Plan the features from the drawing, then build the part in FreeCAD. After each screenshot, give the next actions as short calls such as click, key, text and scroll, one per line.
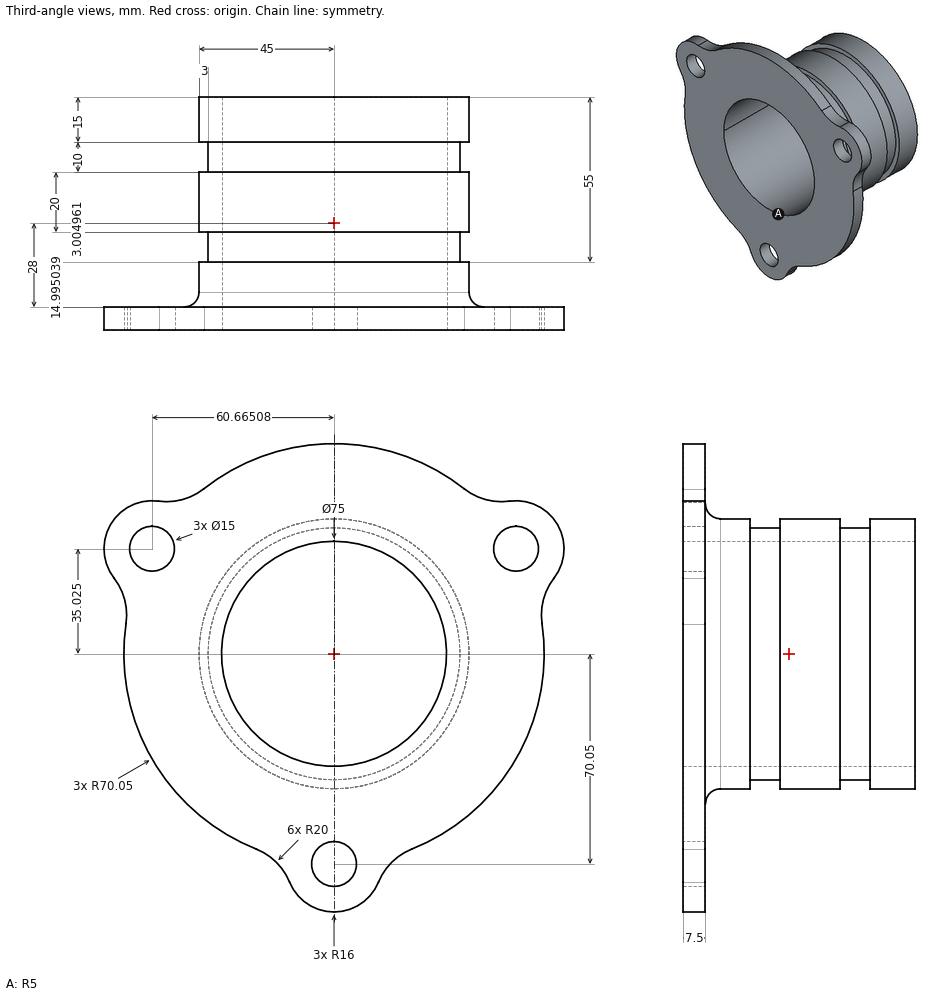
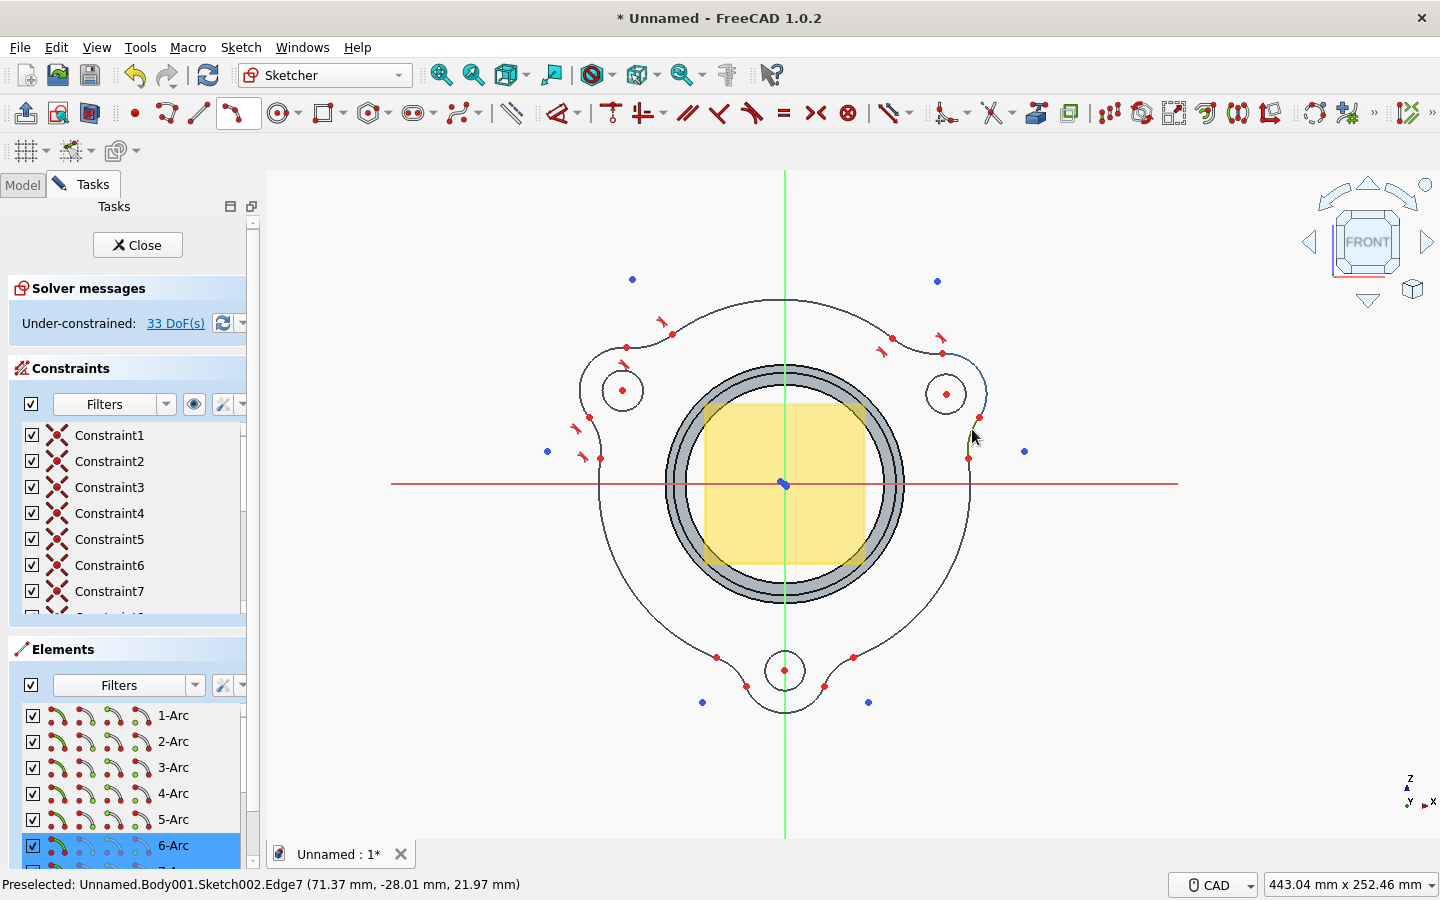
key(t)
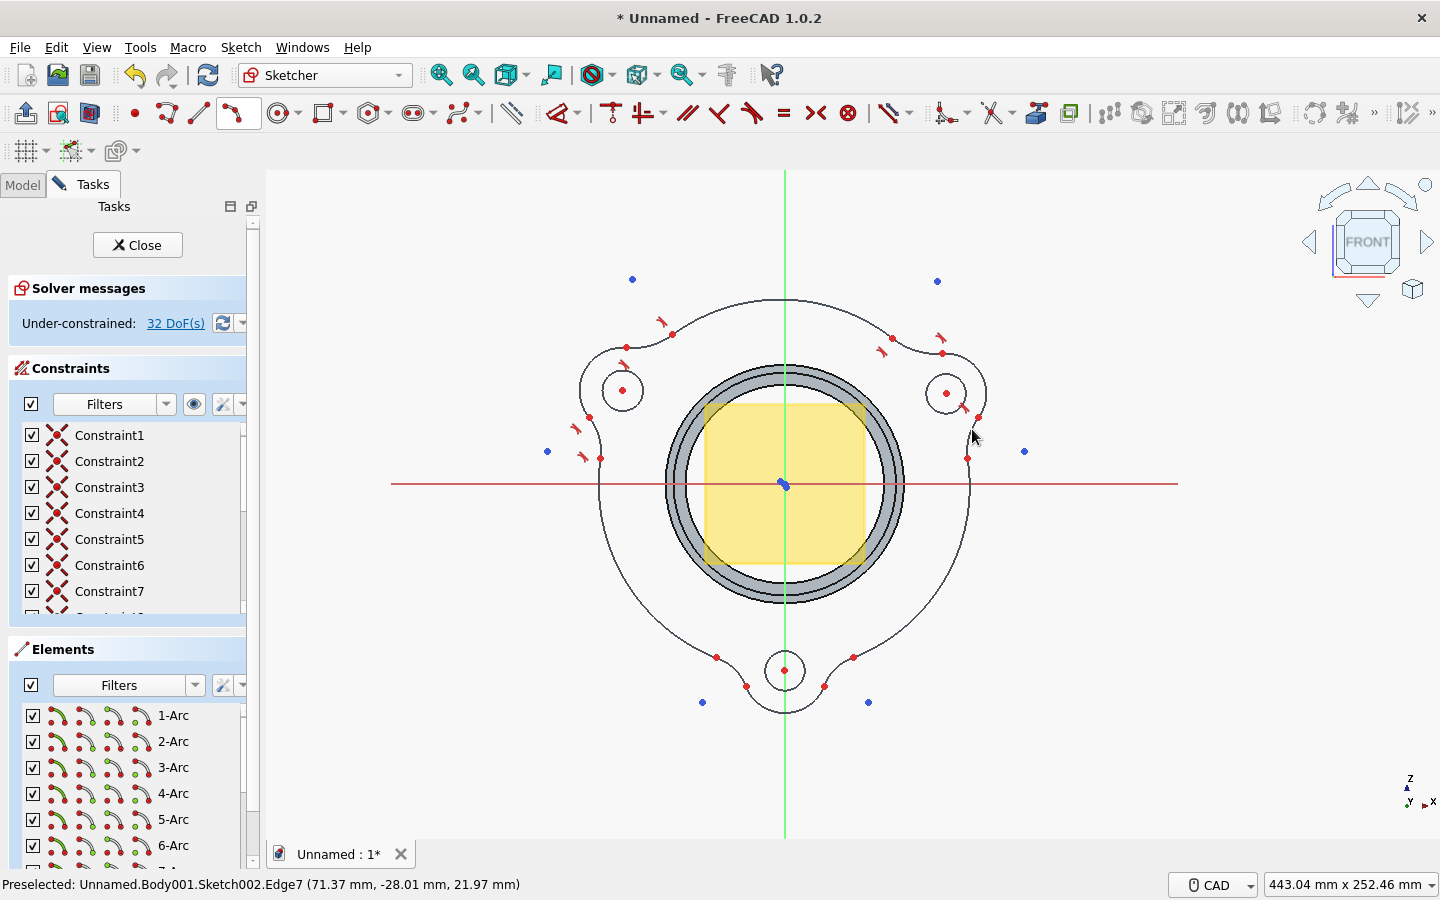
click(972, 429)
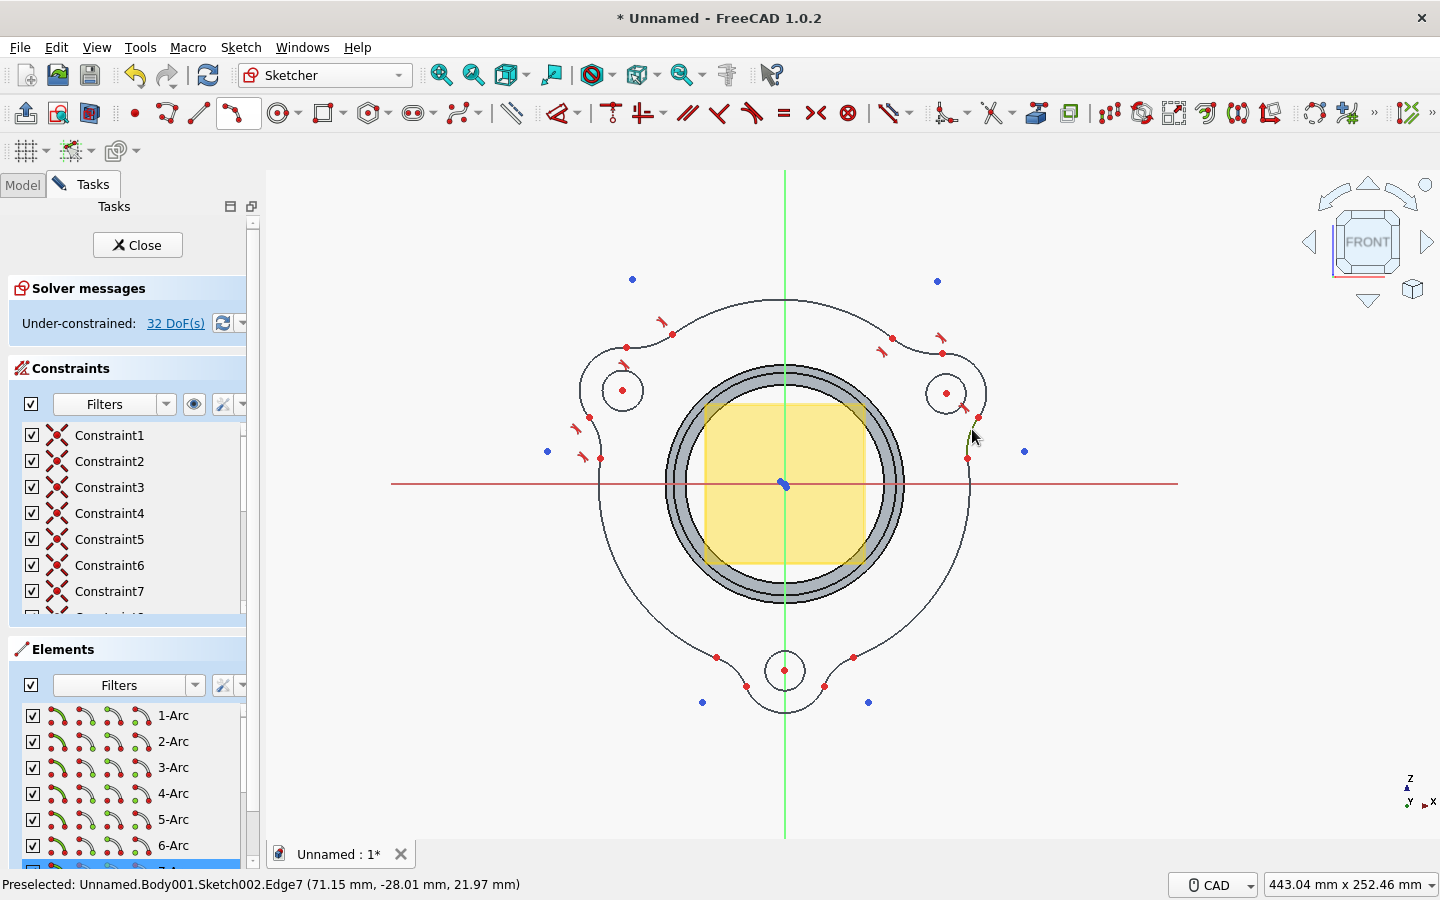
click(915, 618)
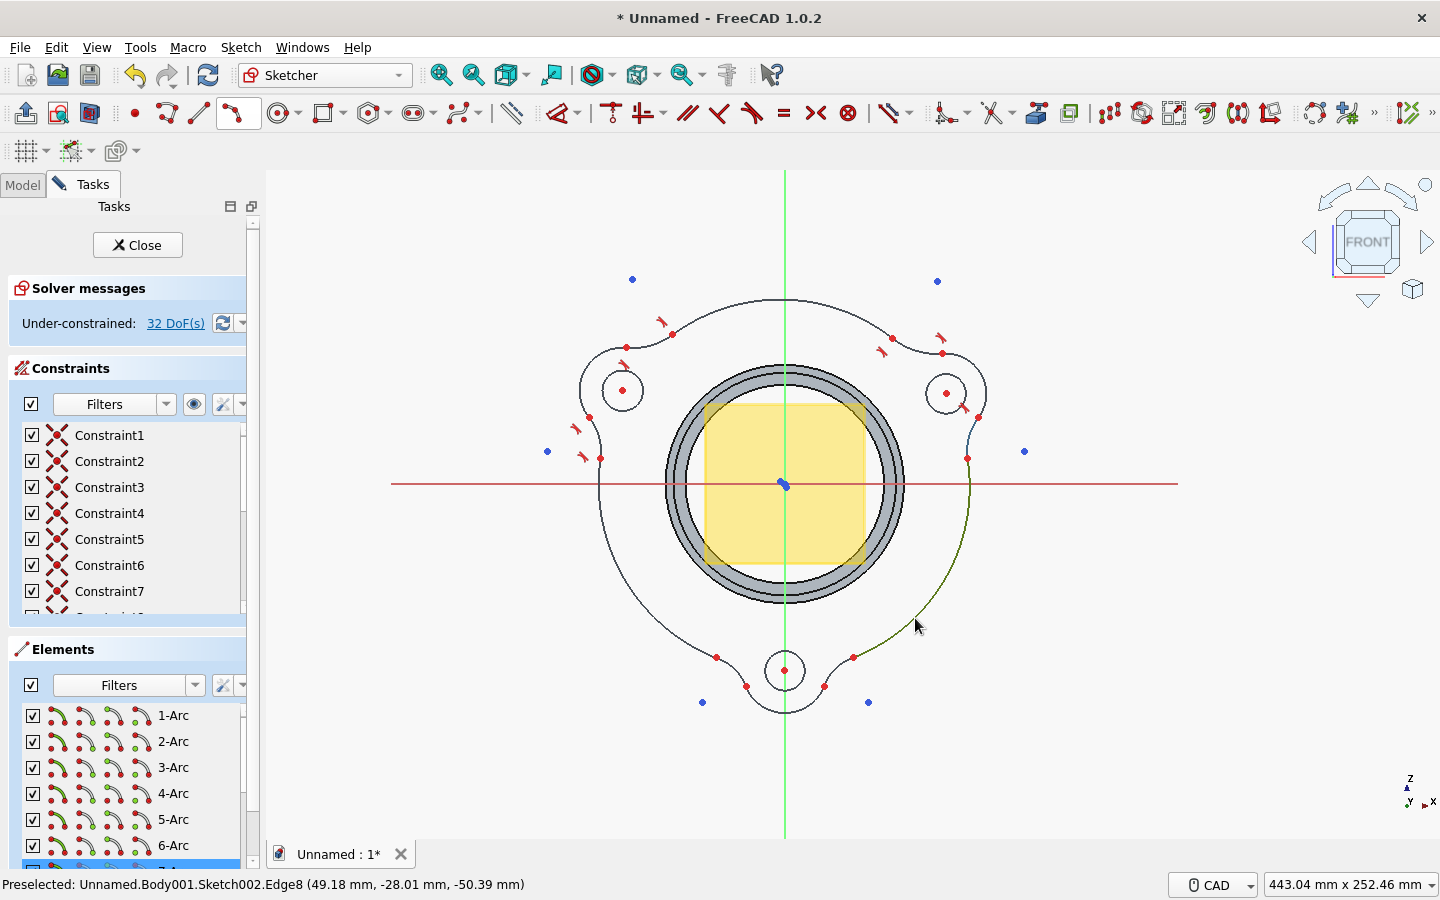
click(752, 114)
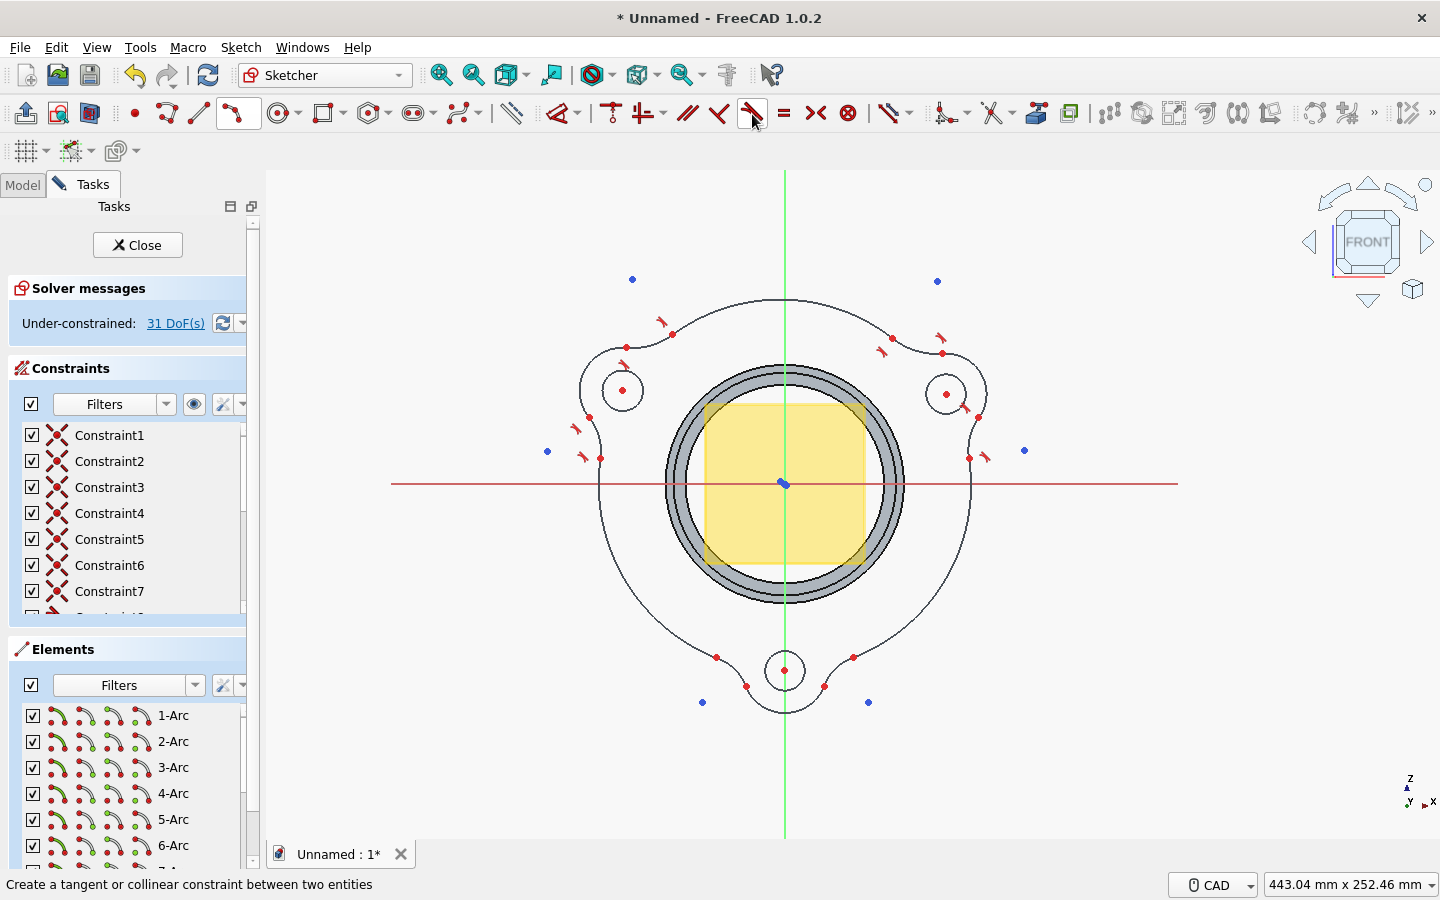
click(915, 618)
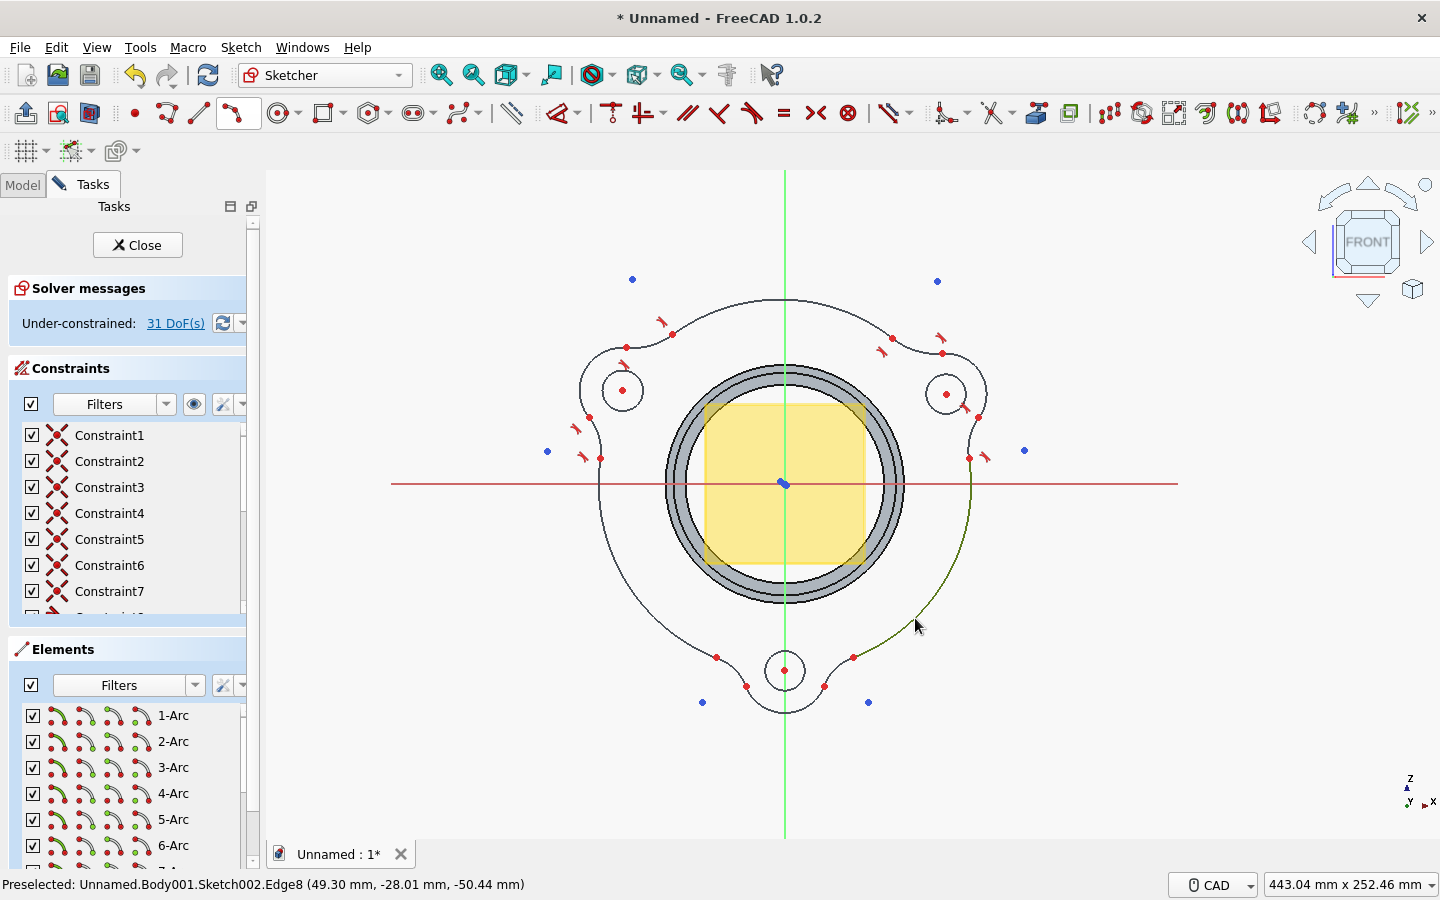
click(842, 664)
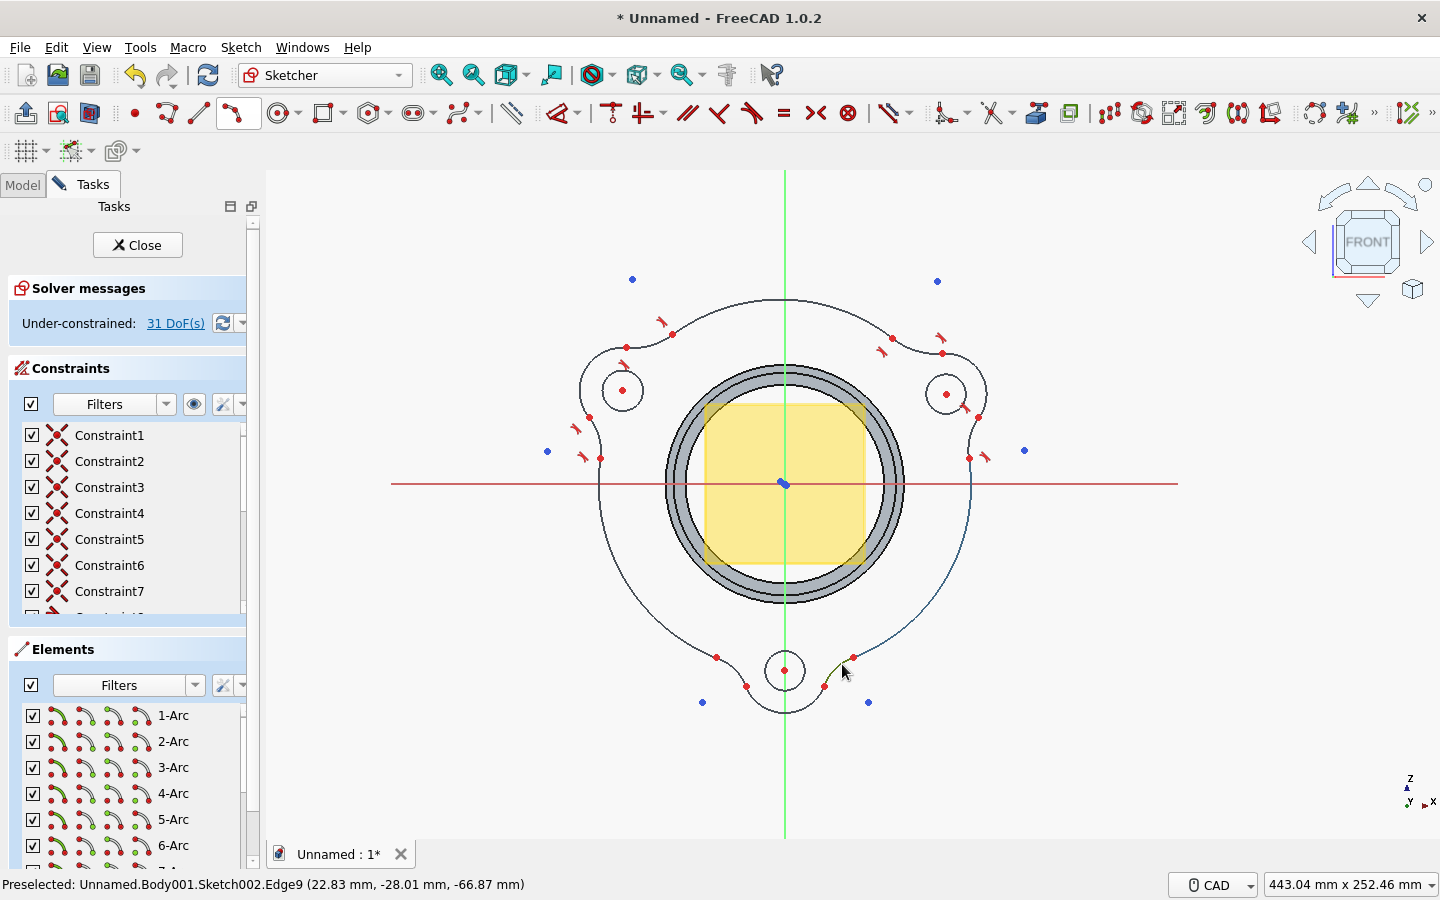
key(t)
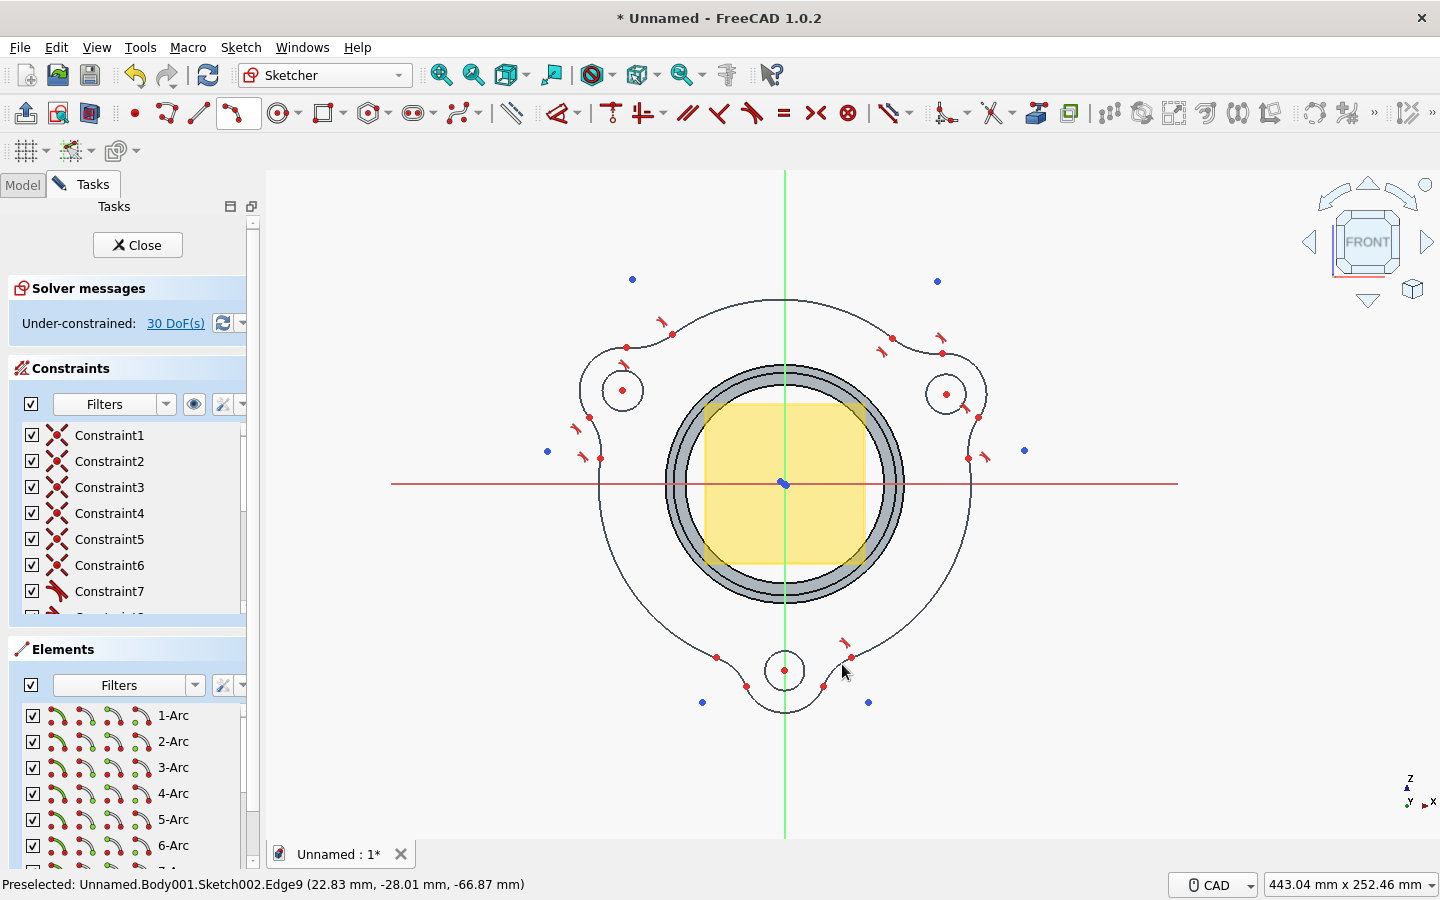
click(841, 664)